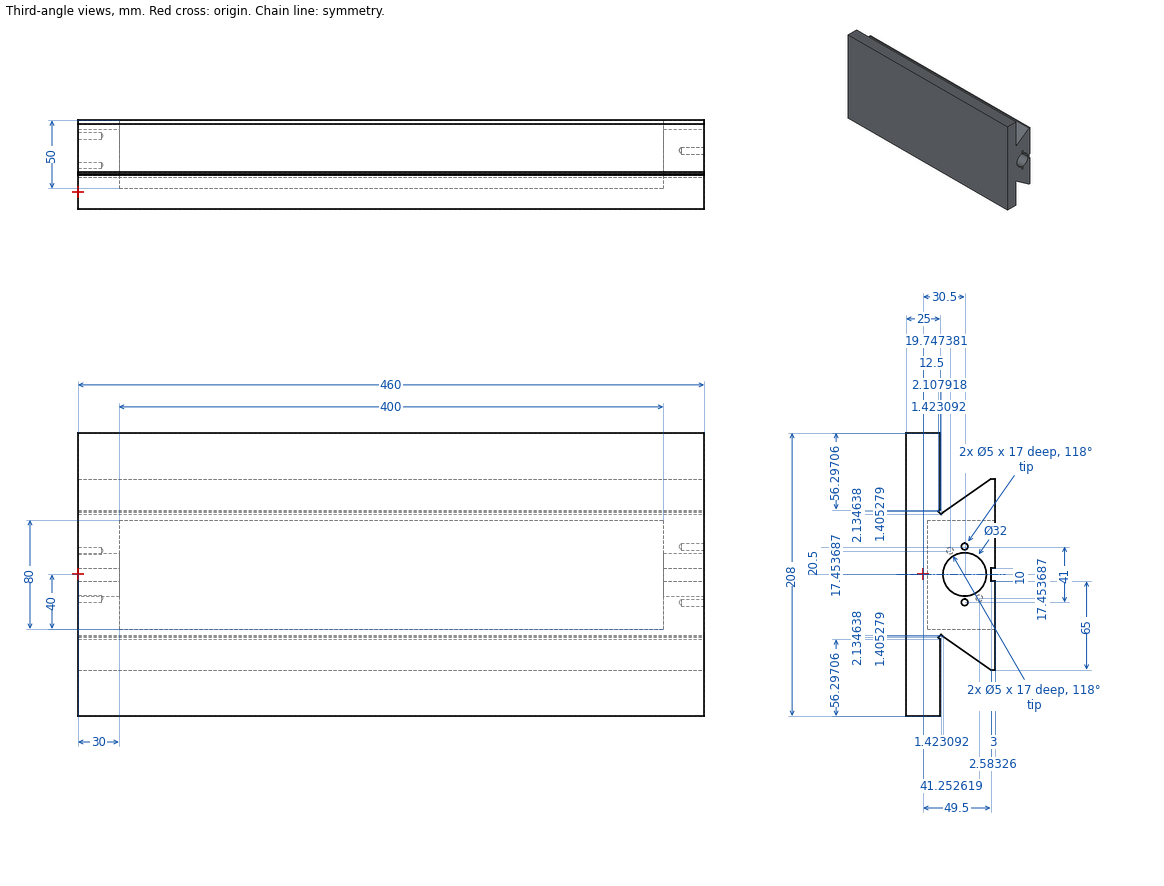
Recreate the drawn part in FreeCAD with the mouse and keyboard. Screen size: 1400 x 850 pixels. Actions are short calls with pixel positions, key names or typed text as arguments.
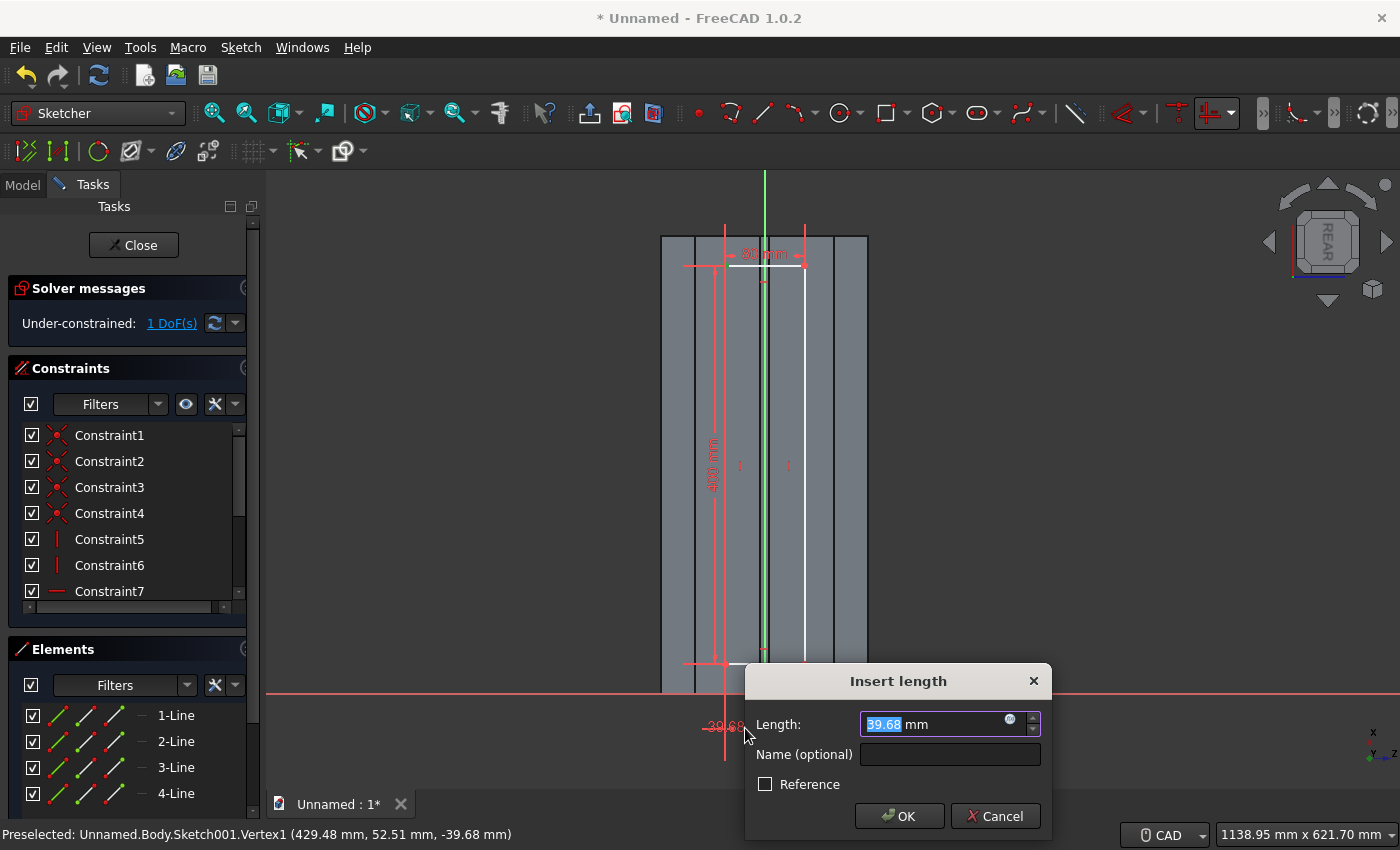
text(40)
key(Return)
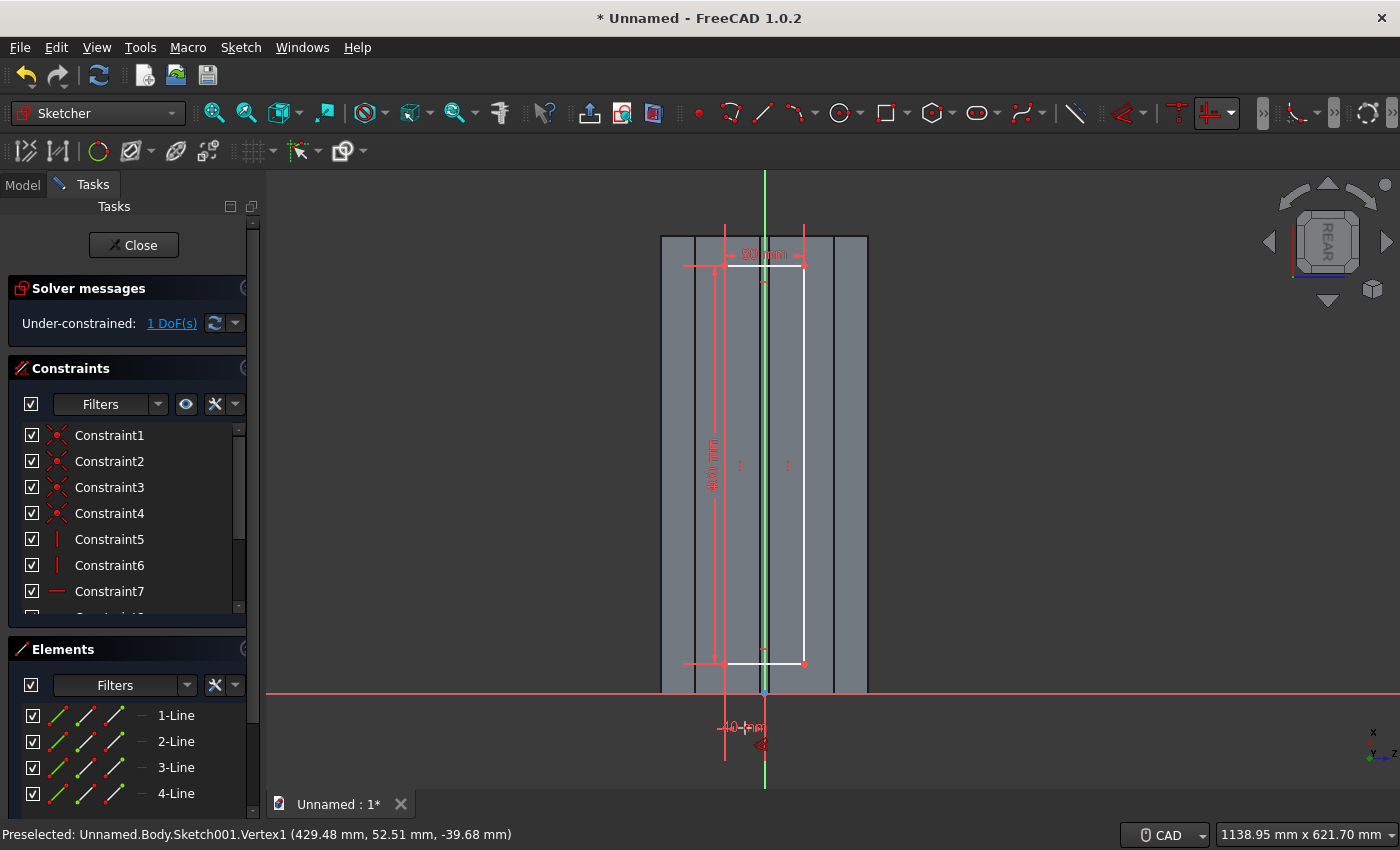
scroll(725, 664, up, 2)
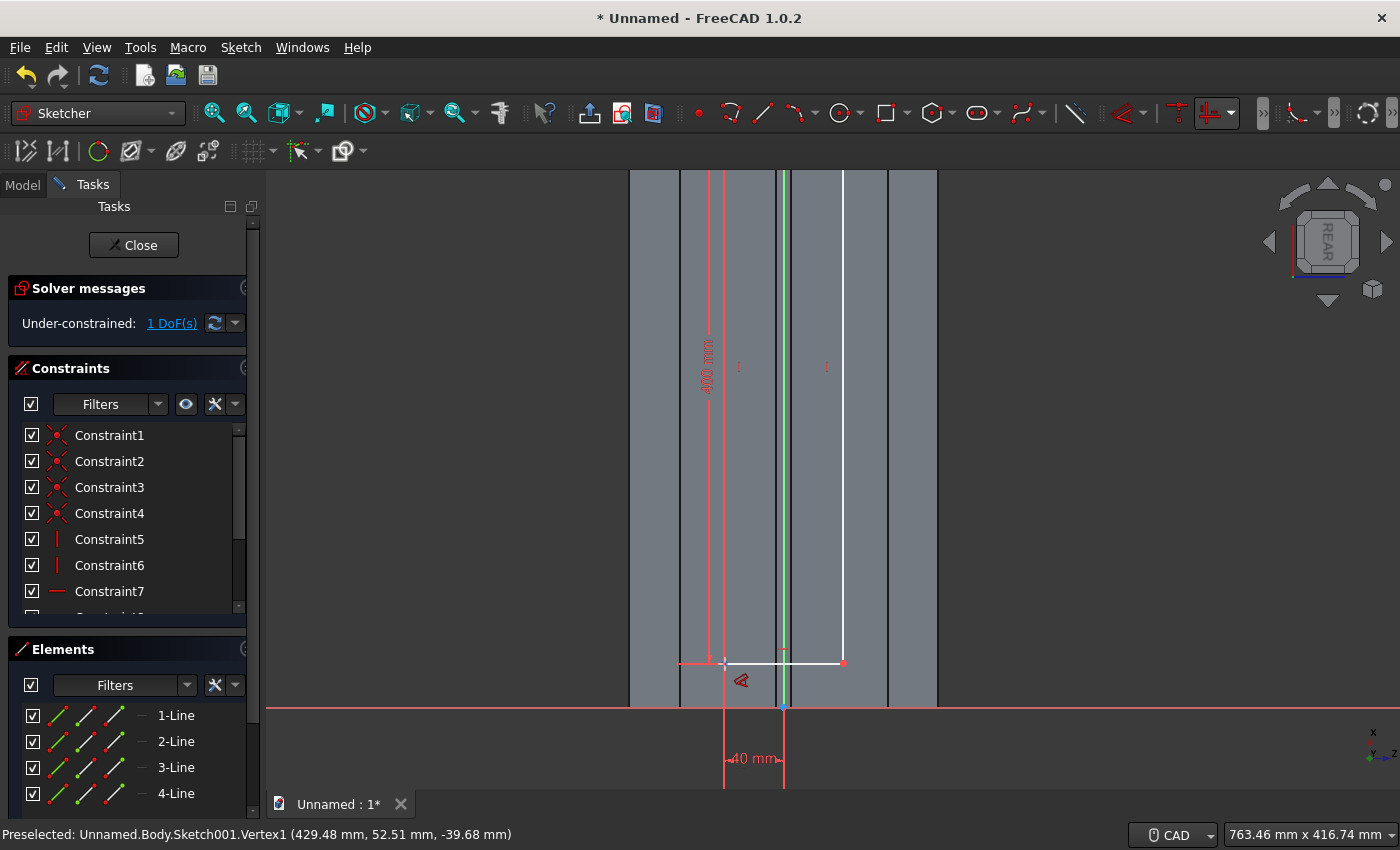
click(724, 664)
click(690, 686)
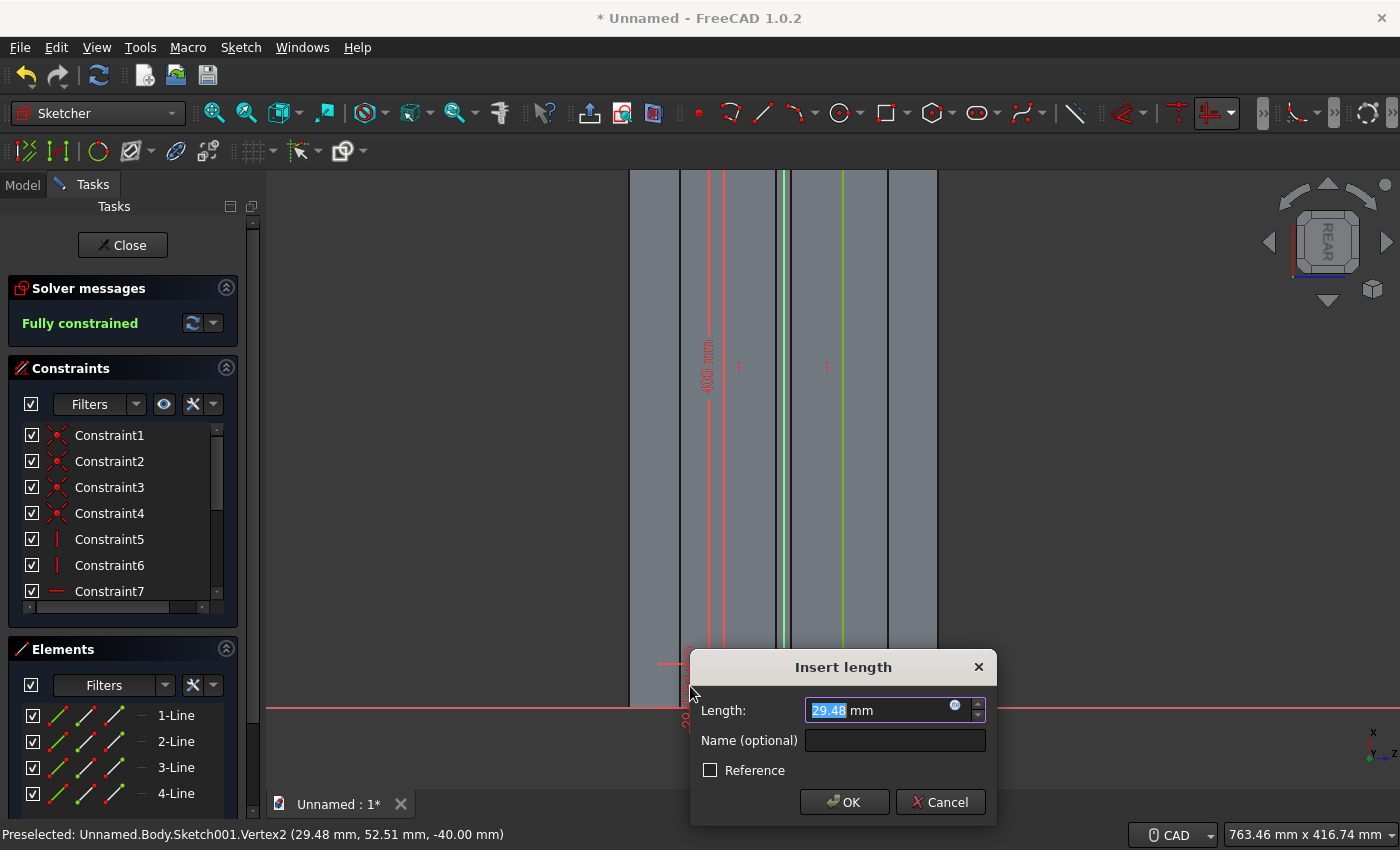
text(30)
key(Return)
key(Escape)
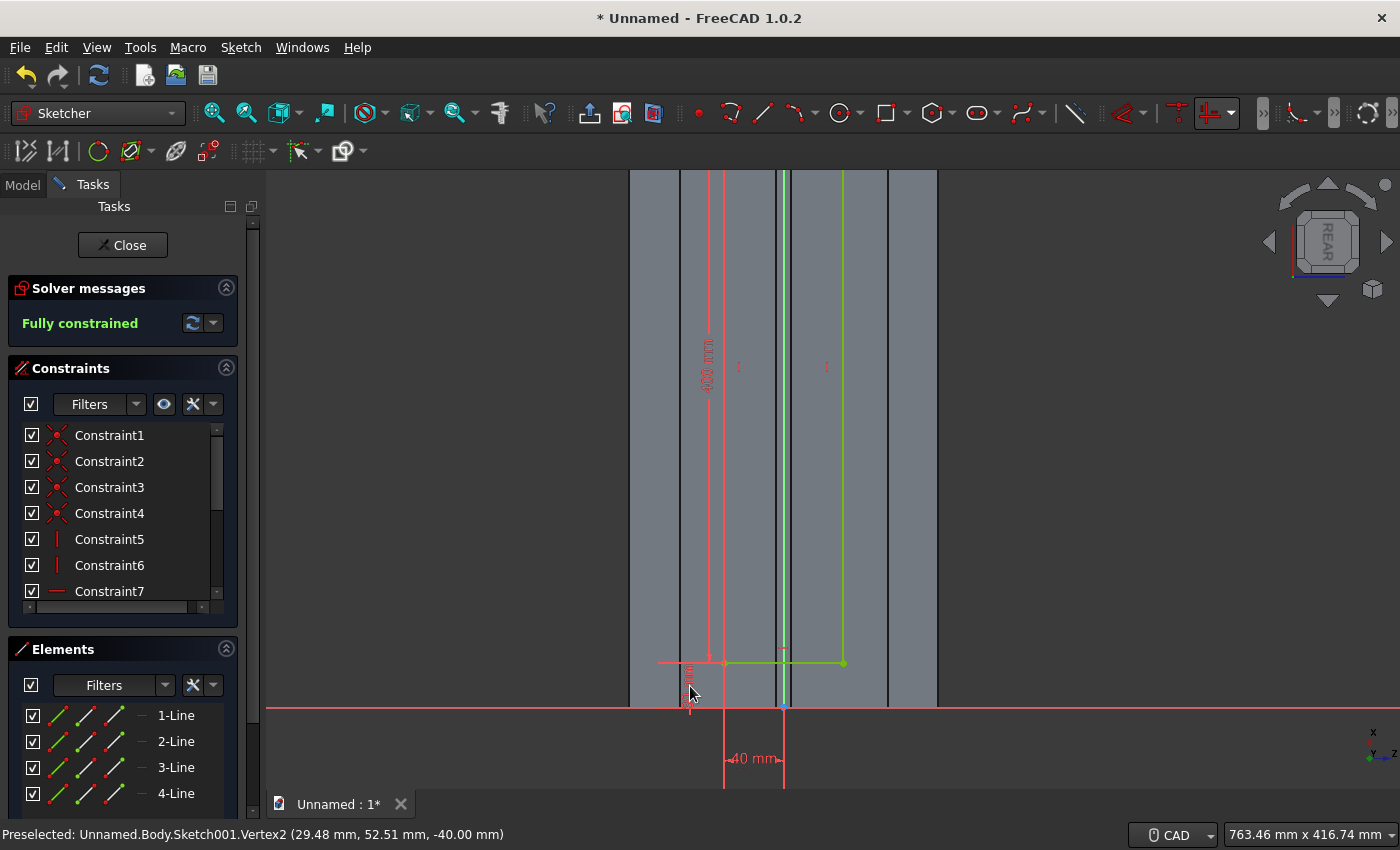
click(123, 245)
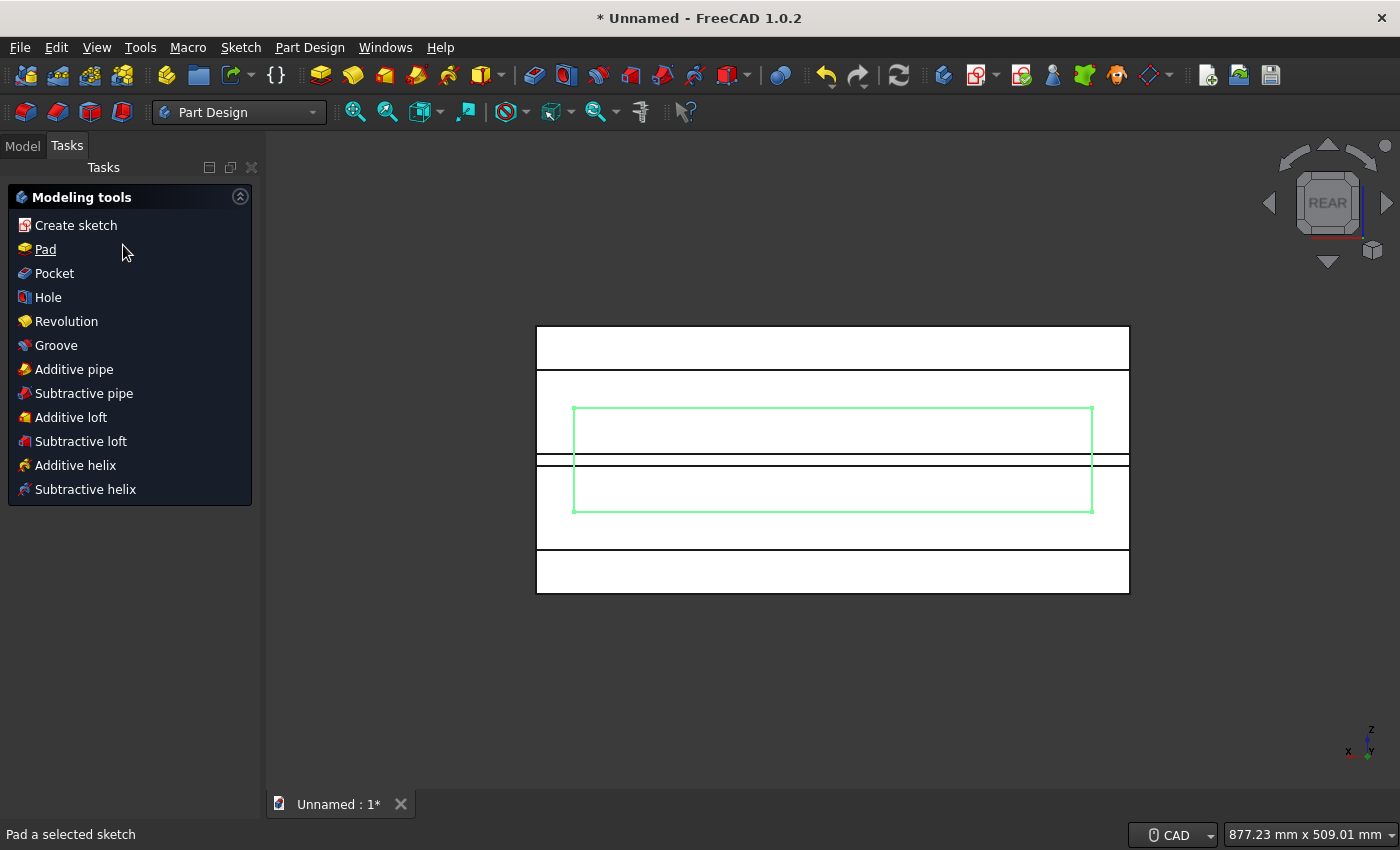
click(536, 76)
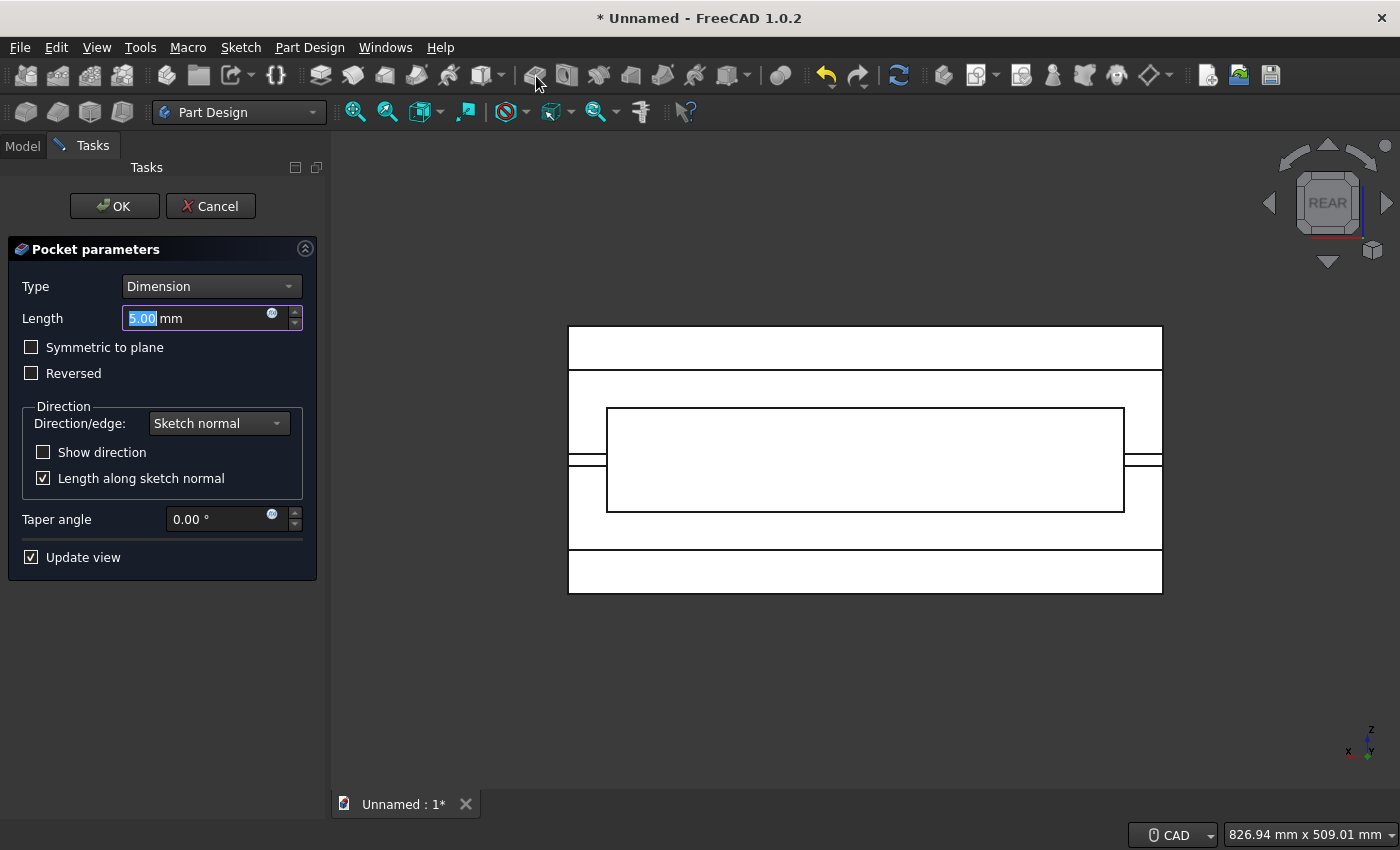
text(50)
key(Tab)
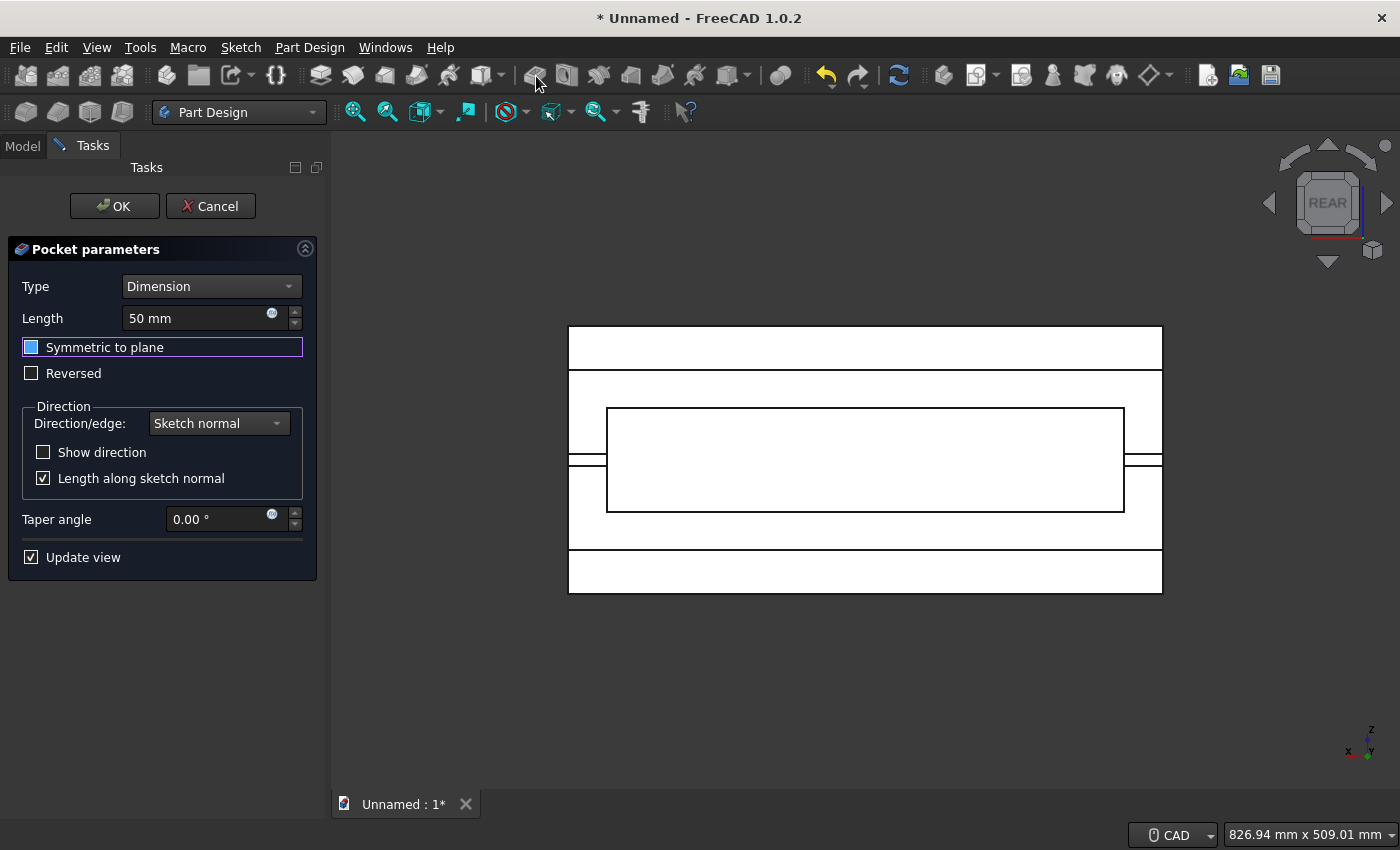
click(115, 206)